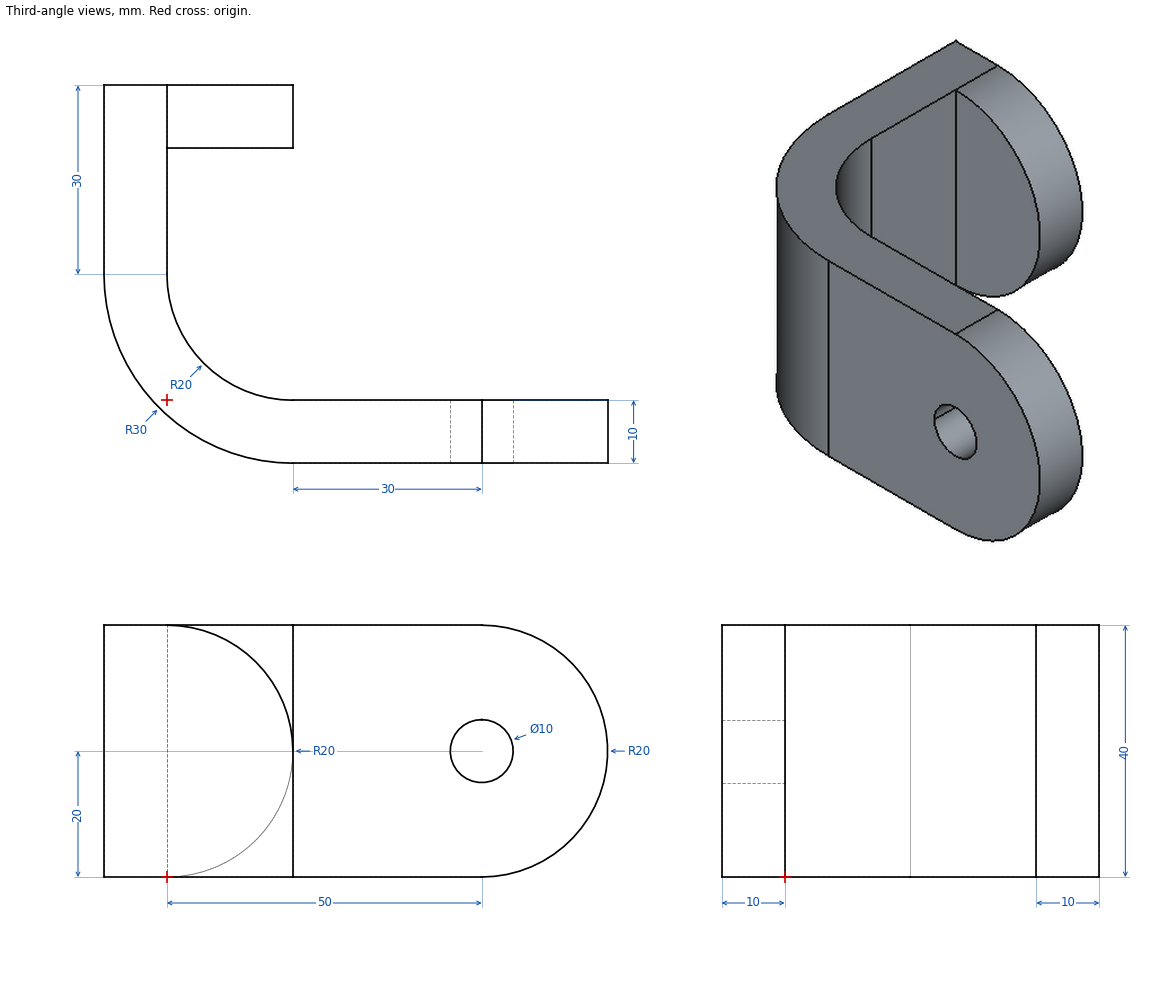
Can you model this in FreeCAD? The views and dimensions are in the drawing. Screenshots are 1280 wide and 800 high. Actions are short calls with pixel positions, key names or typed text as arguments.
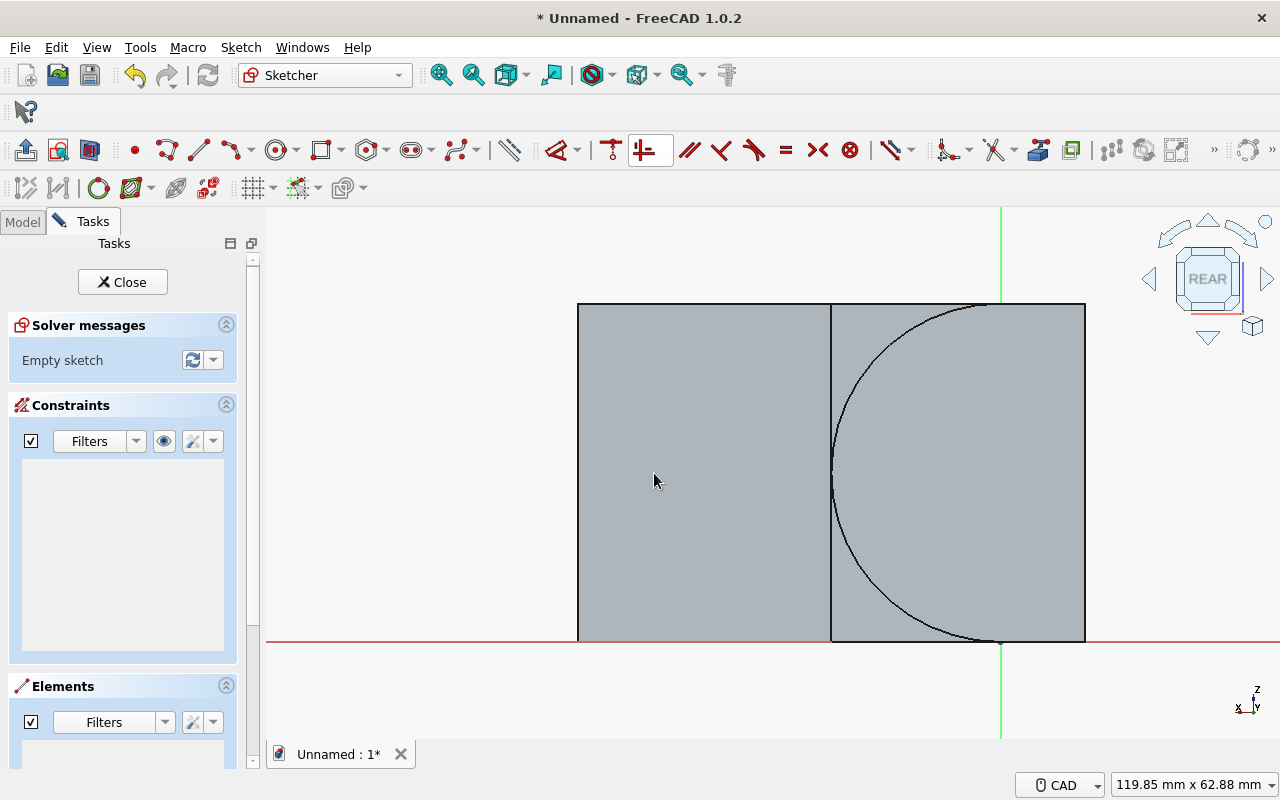
key(g)
key(l)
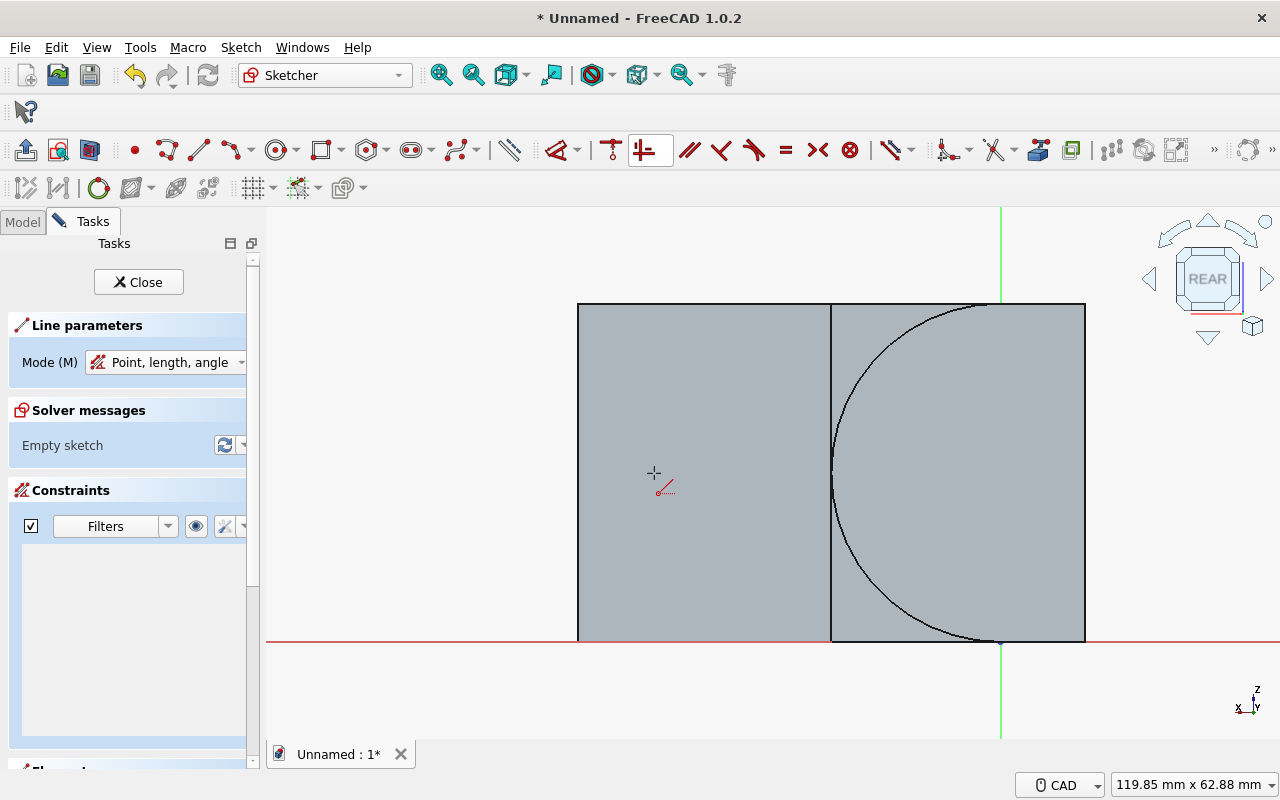
click(578, 642)
click(578, 304)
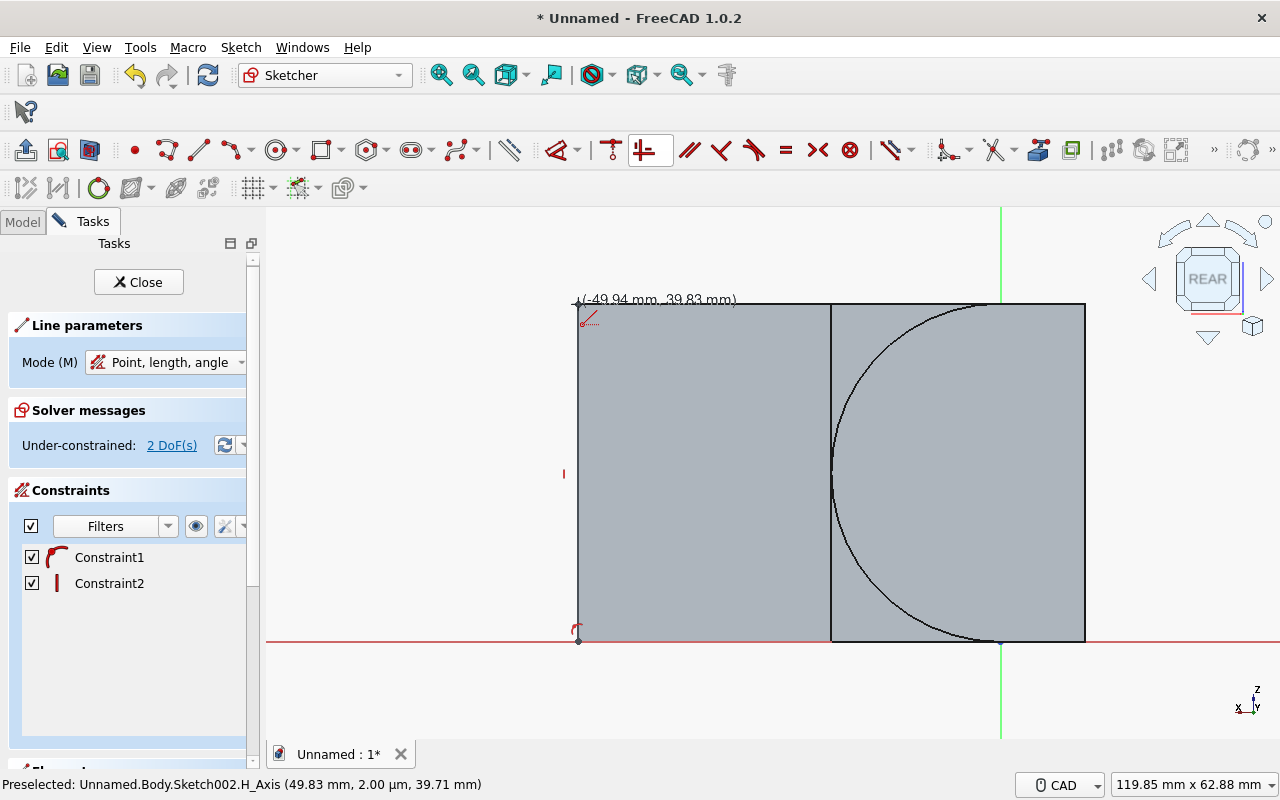
key(g)
key(3)
key(a)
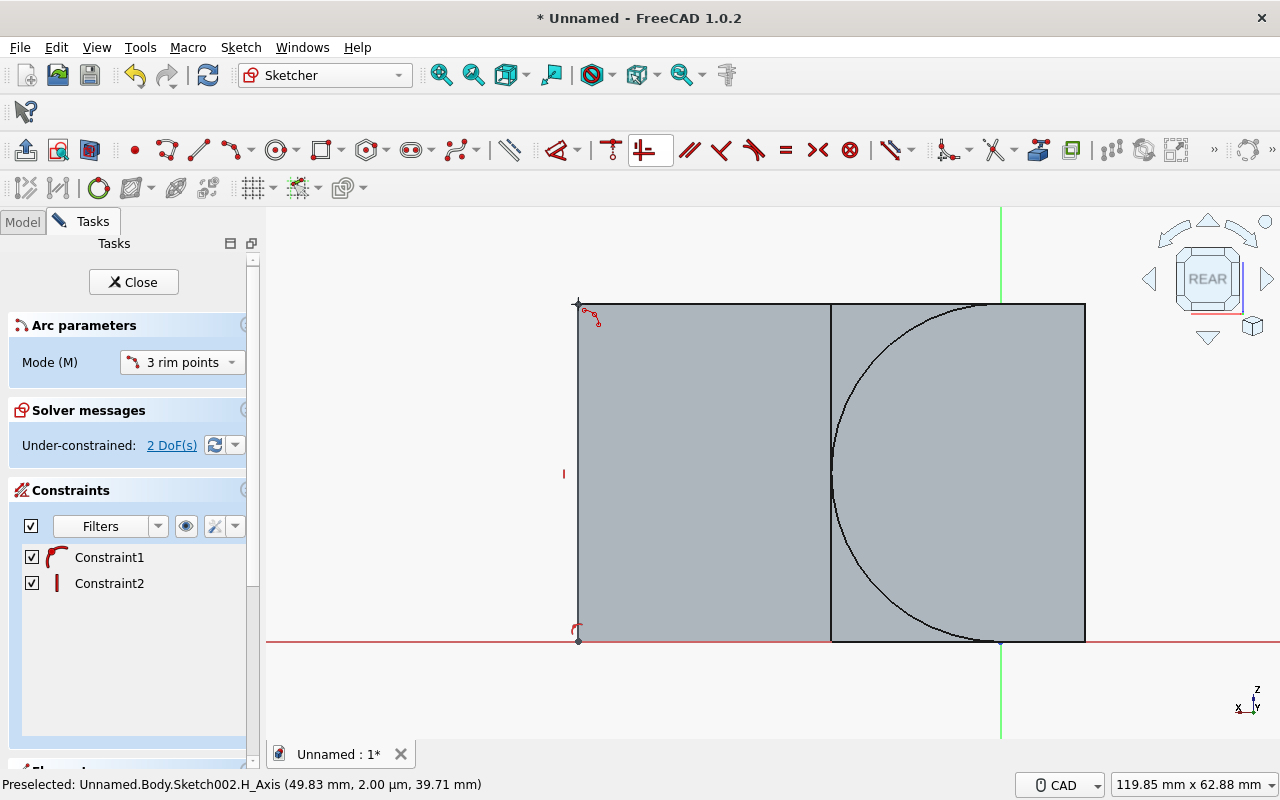
click(578, 305)
click(578, 642)
click(408, 473)
key(Escape)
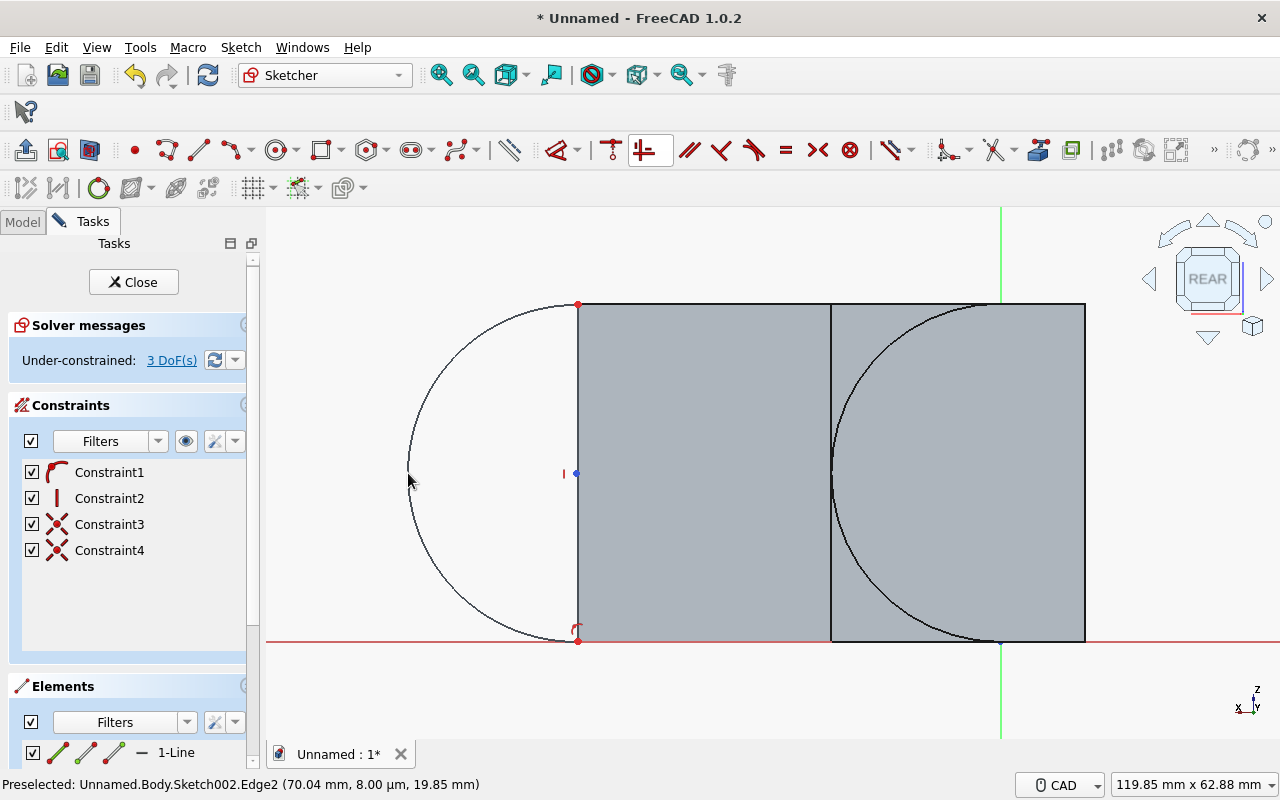
key(d)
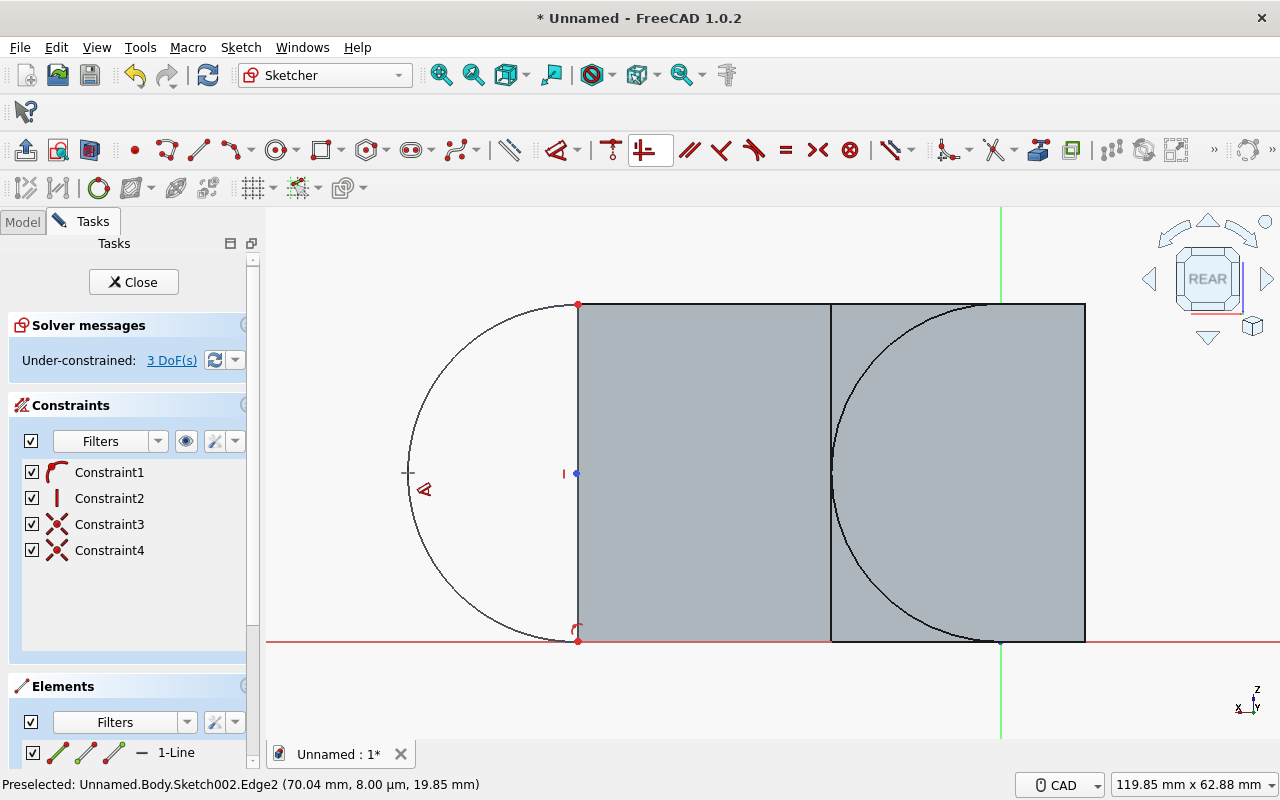
click(441, 374)
click(415, 355)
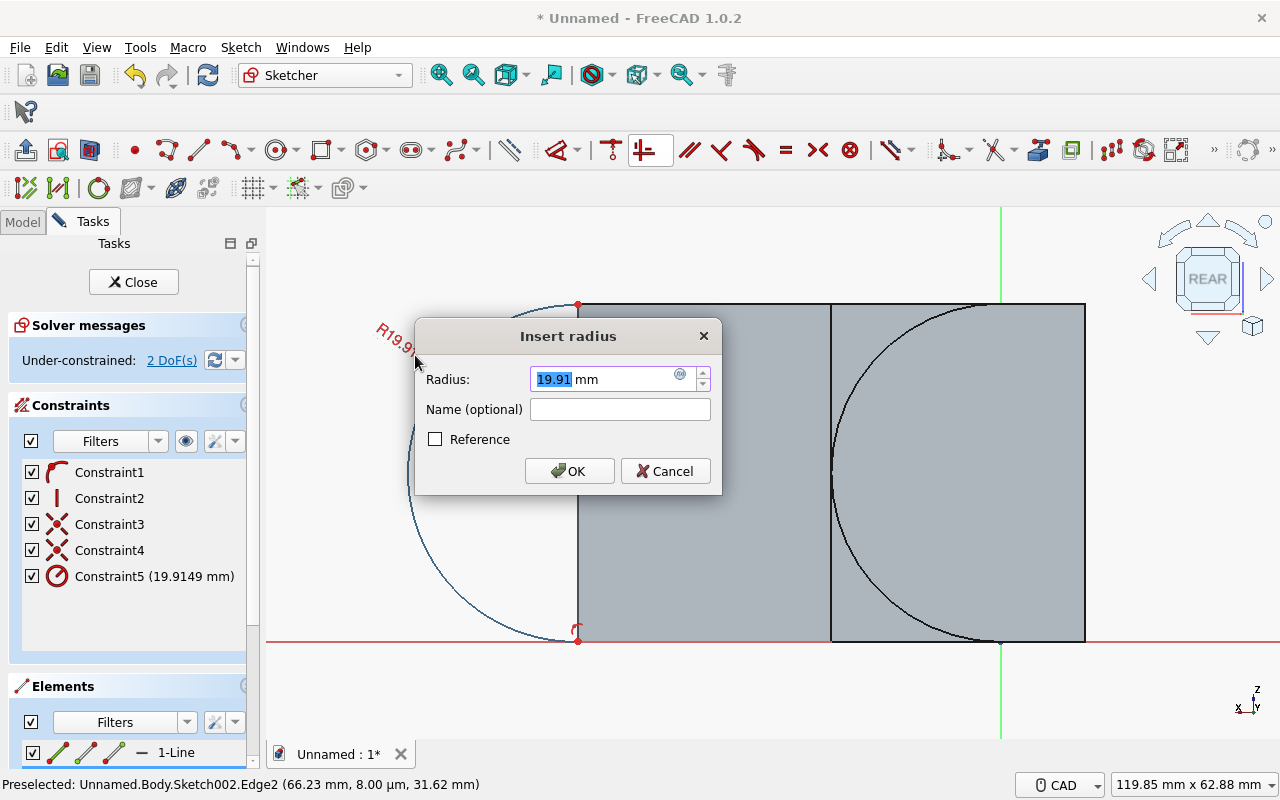
text(20)
key(Return)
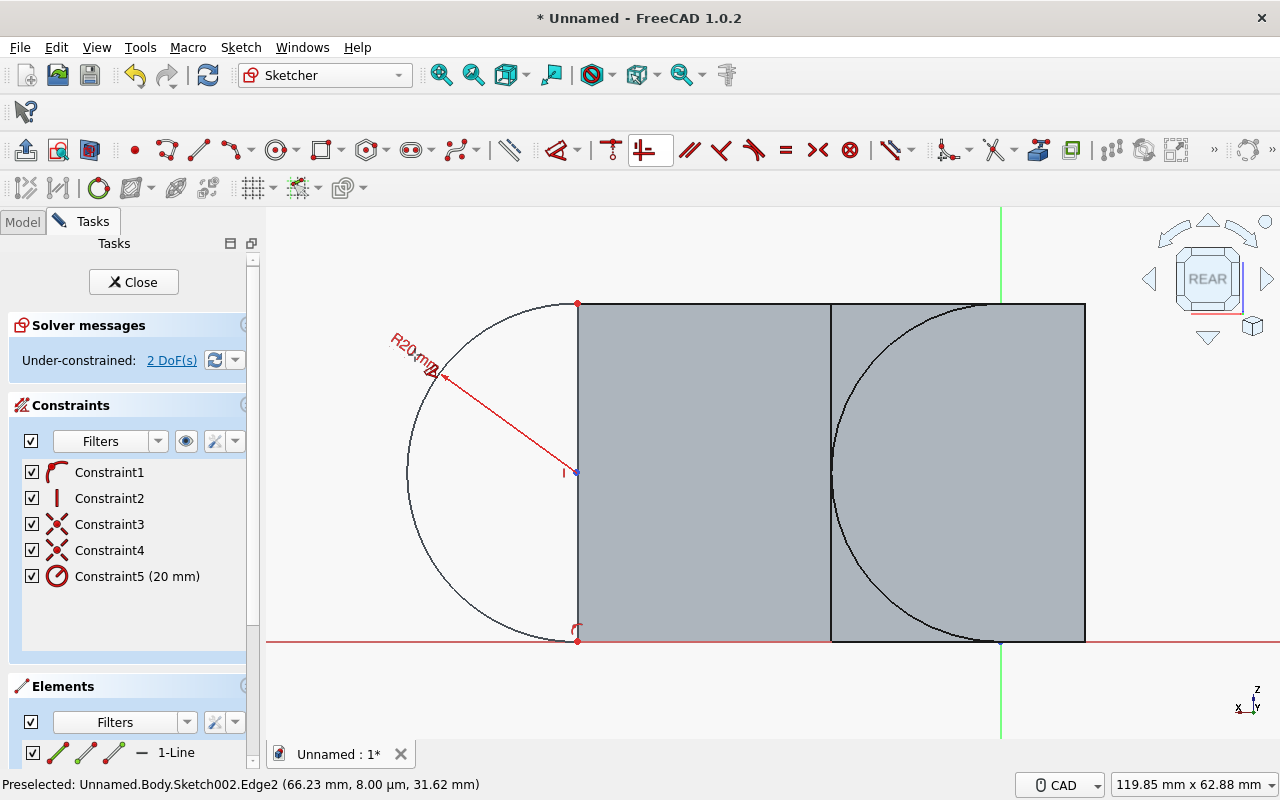
click(578, 642)
click(789, 676)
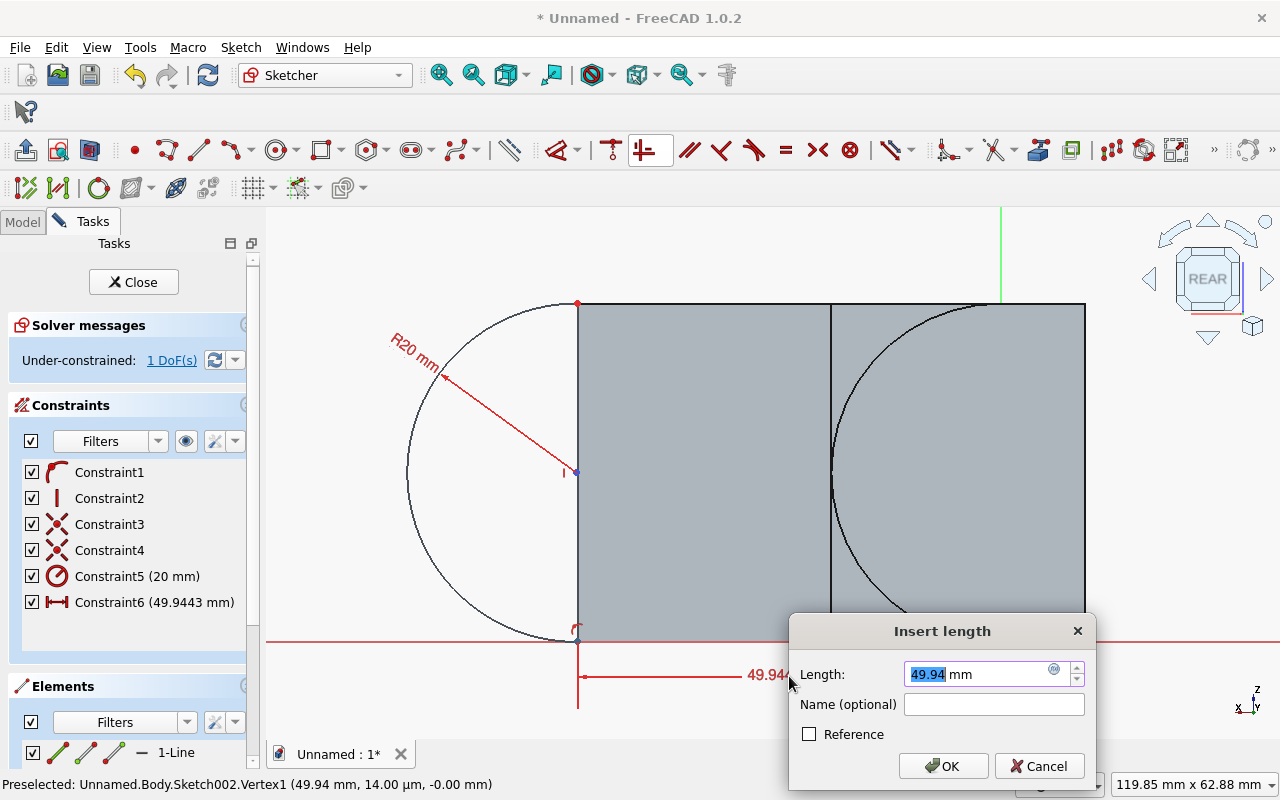
text(50)
key(Return)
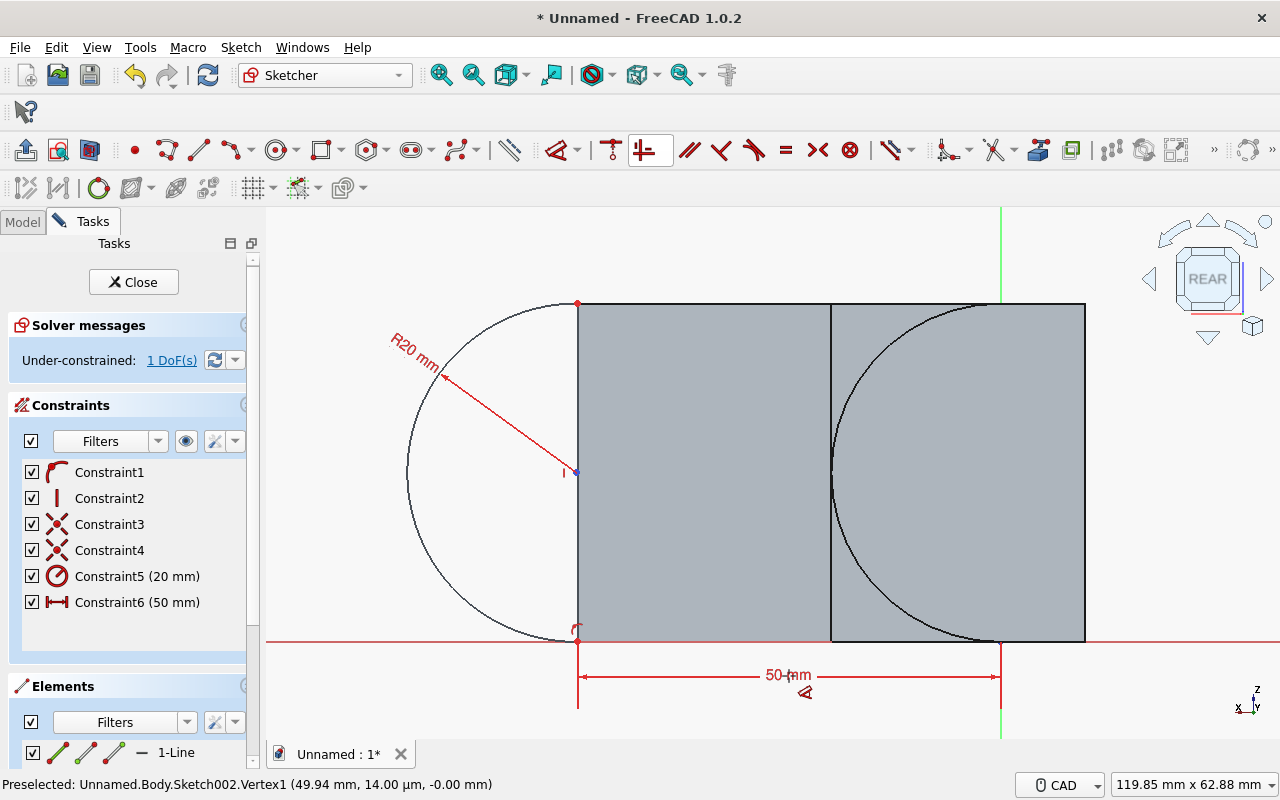
click(576, 473)
click(691, 676)